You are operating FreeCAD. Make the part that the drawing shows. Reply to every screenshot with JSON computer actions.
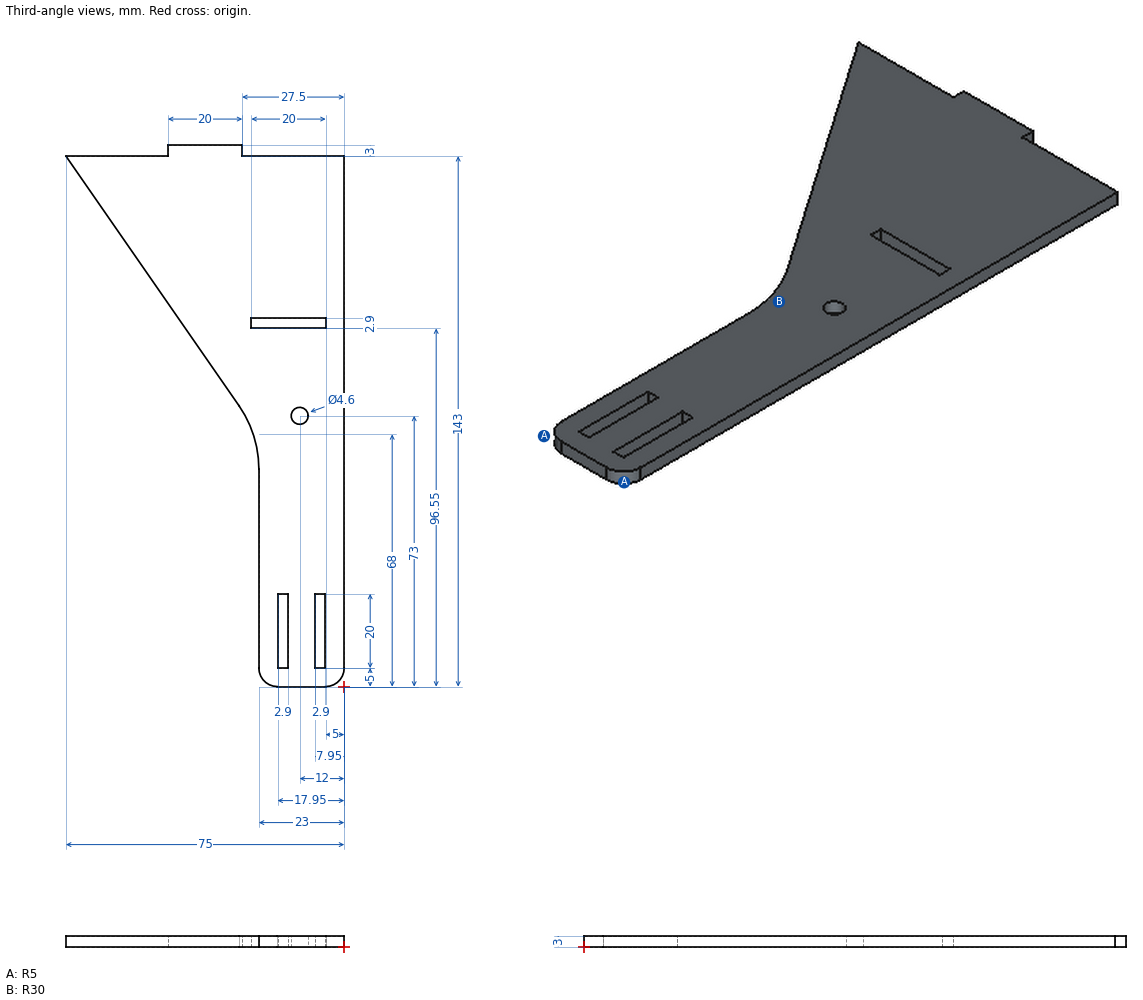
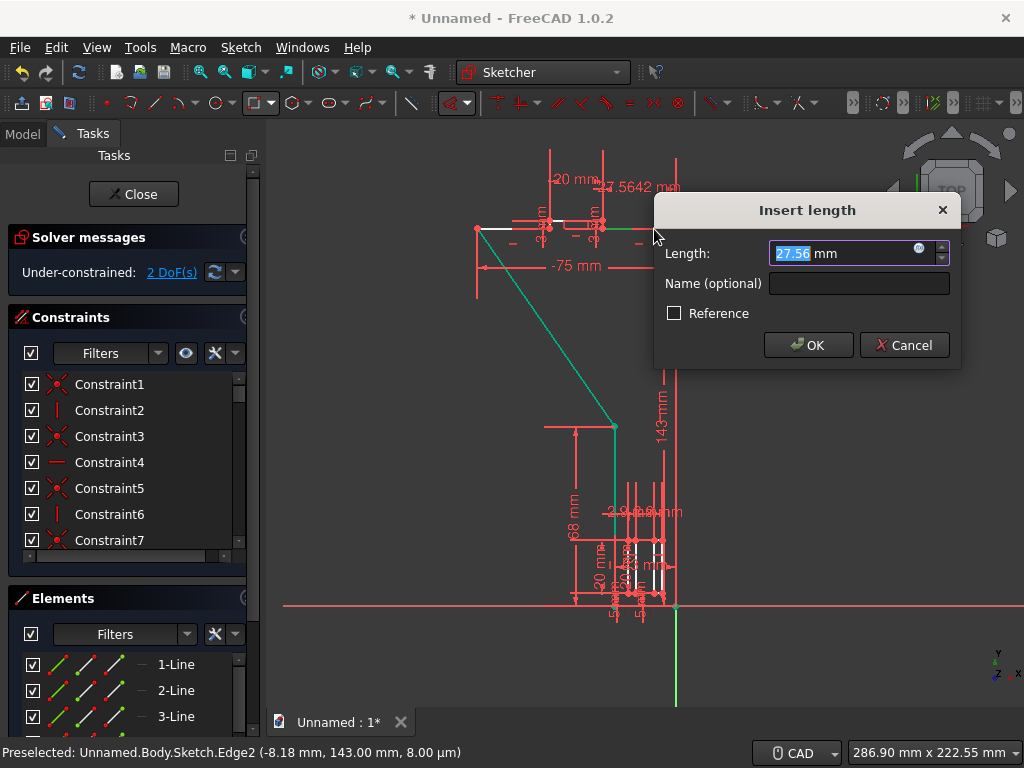
{"action": "type", "text": "27.5"}
{"action": "key", "text": "Return"}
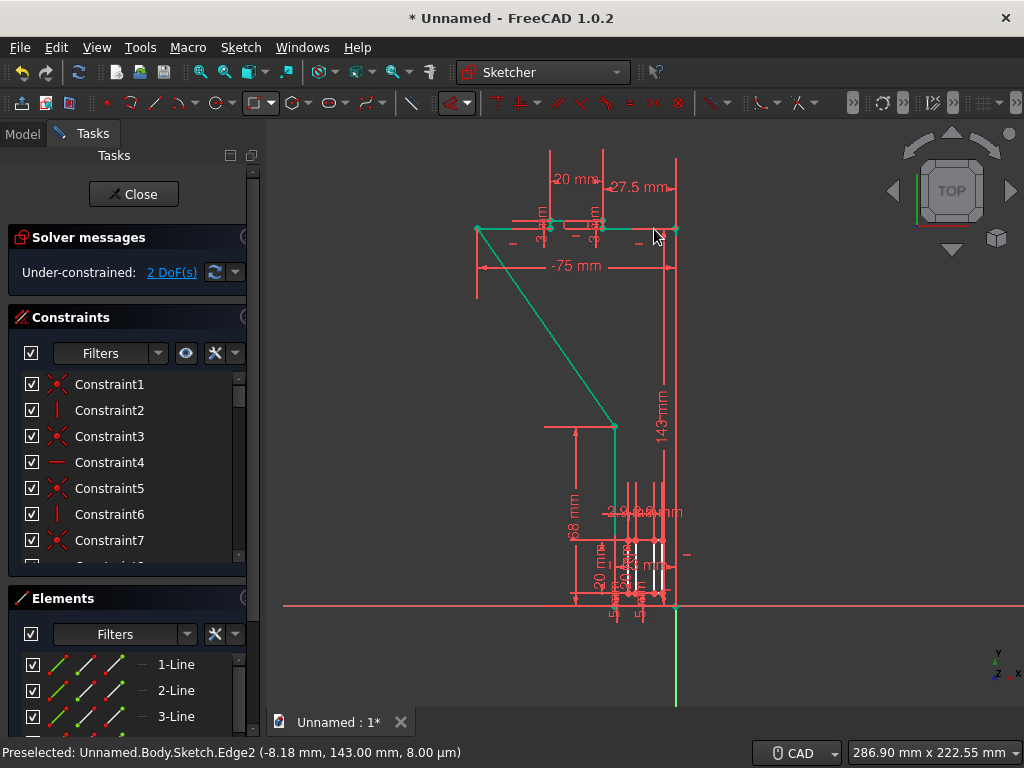
{"action": "scroll", "coordinate": [654, 540], "scroll_direction": "up", "scroll_amount": 4}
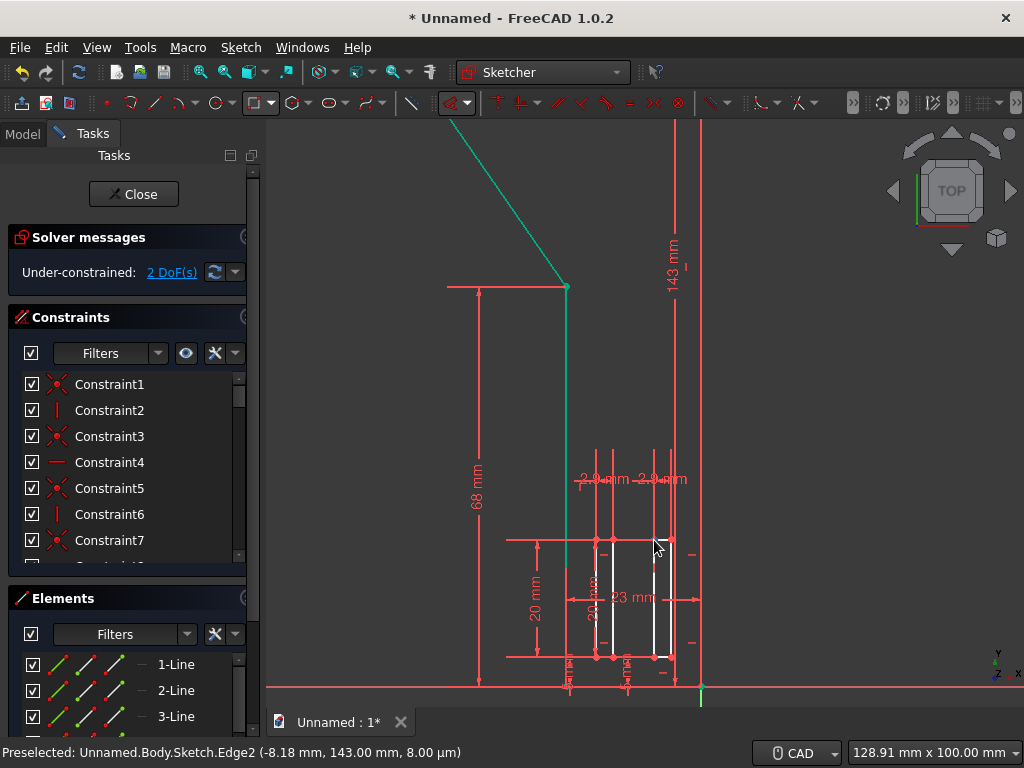
{"action": "left_click", "coordinate": [654, 540]}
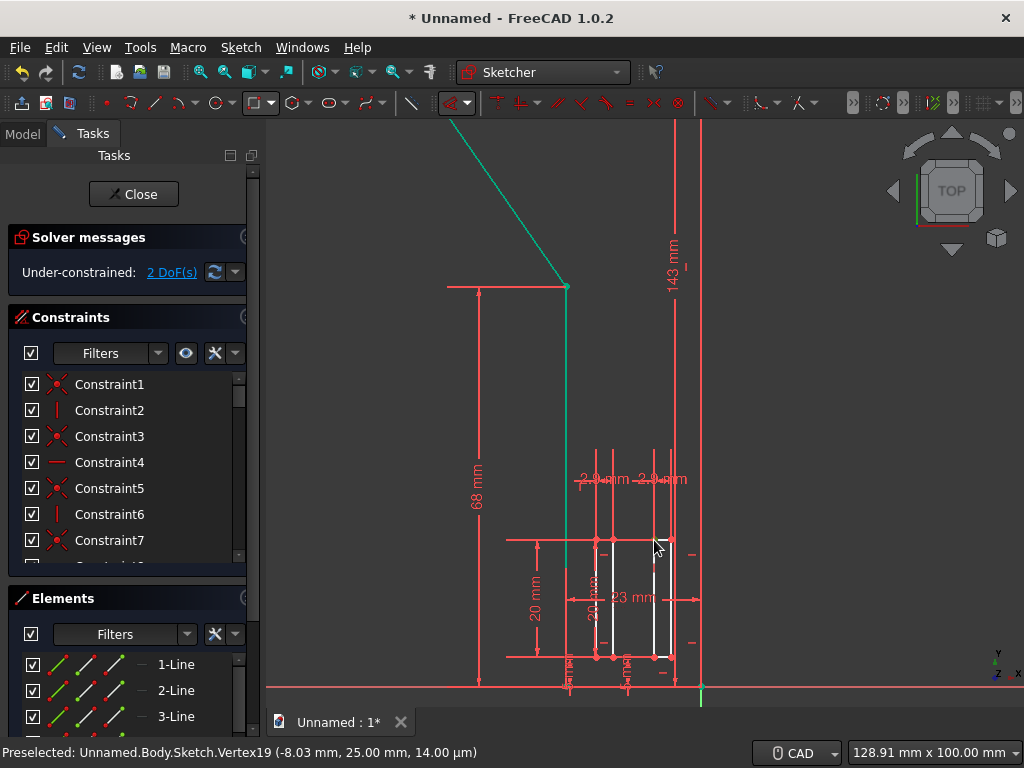
{"action": "key", "text": "l"}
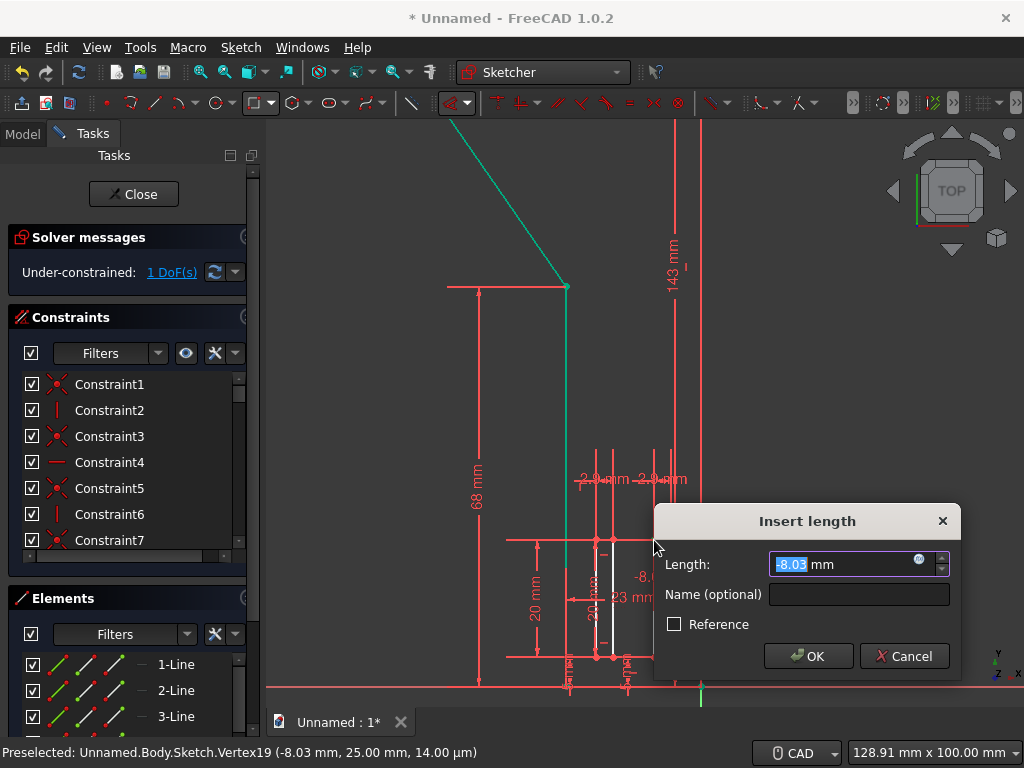
{"action": "type", "text": "-7.95"}
{"action": "key", "text": "Return"}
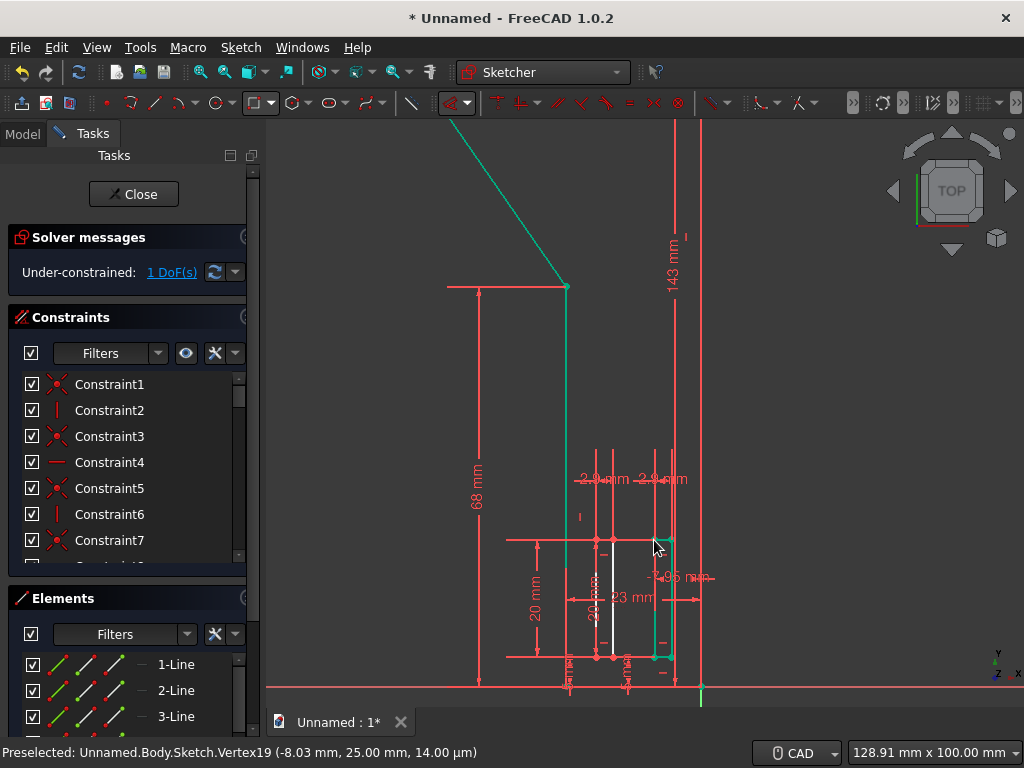
{"action": "left_click", "coordinate": [596, 540]}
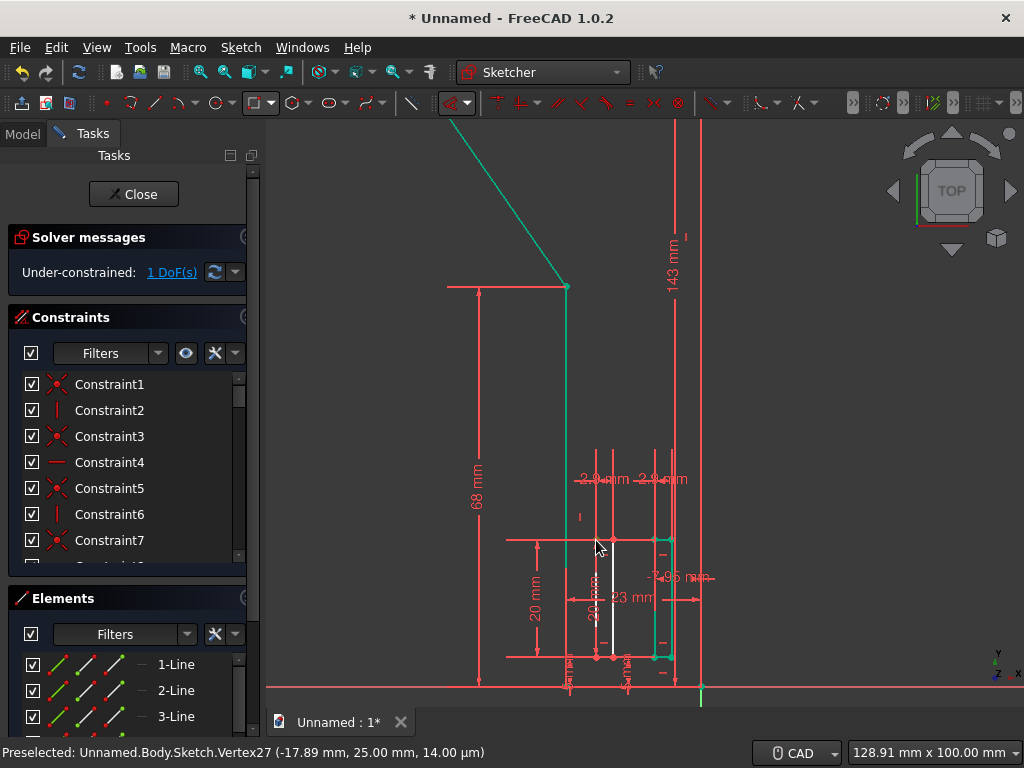
{"action": "left_click", "coordinate": [470, 104]}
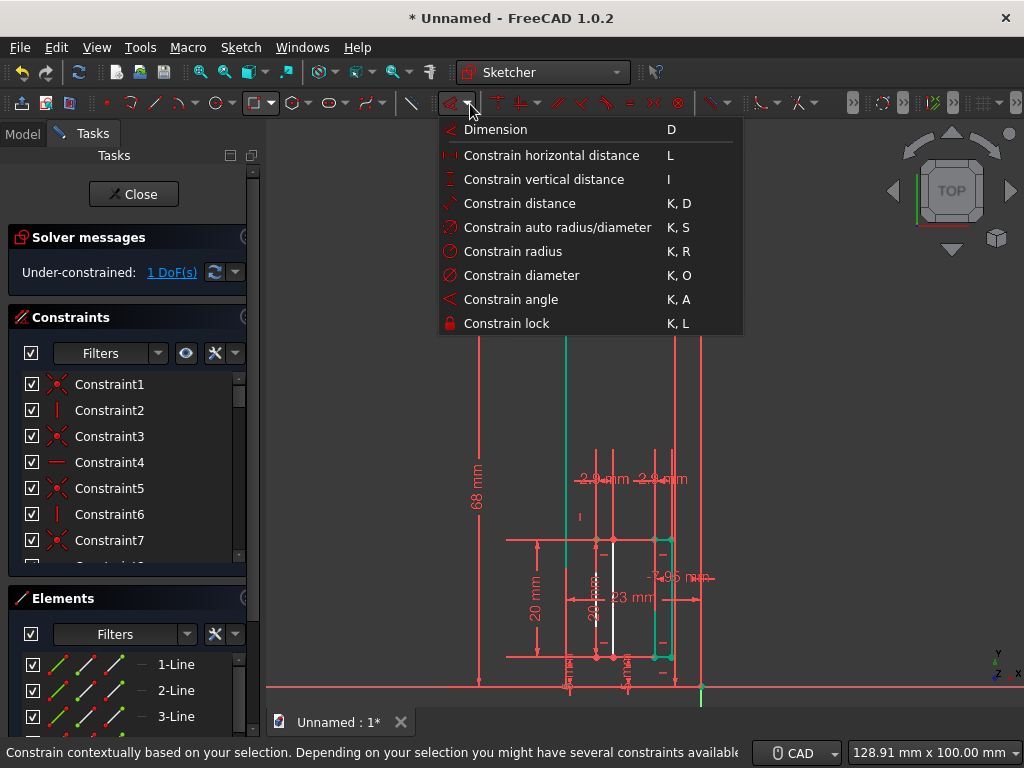
{"action": "left_click", "coordinate": [591, 155]}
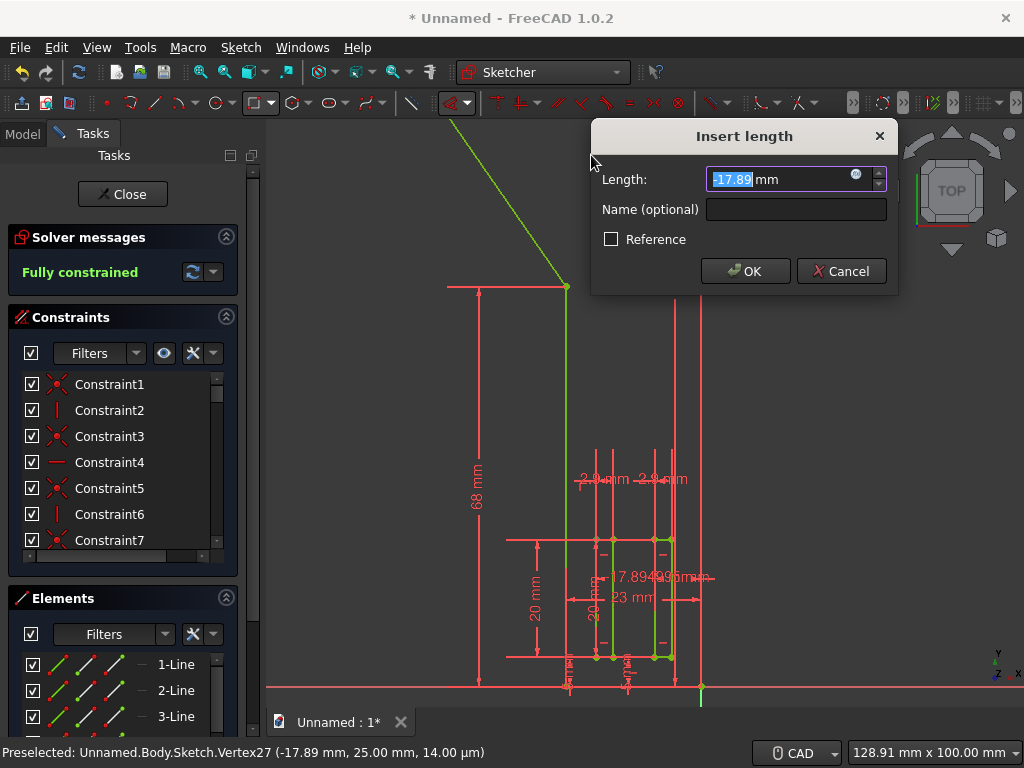
{"action": "type", "text": "-17.95"}
{"action": "key", "text": "Return"}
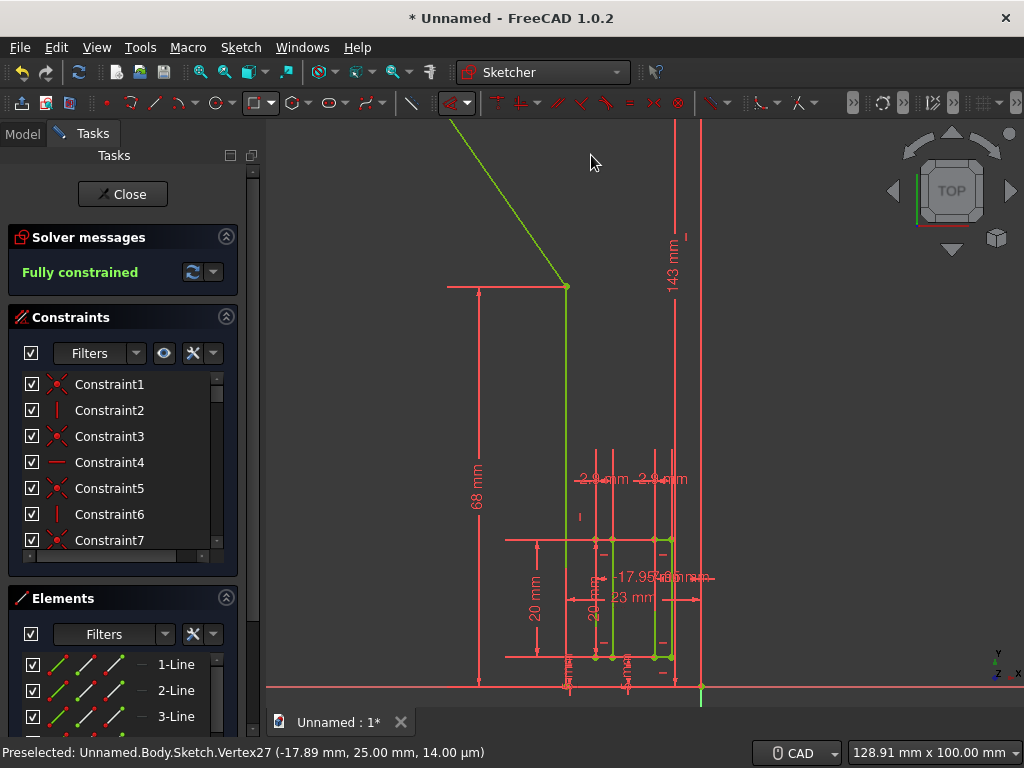
{"action": "left_click", "coordinate": [123, 194]}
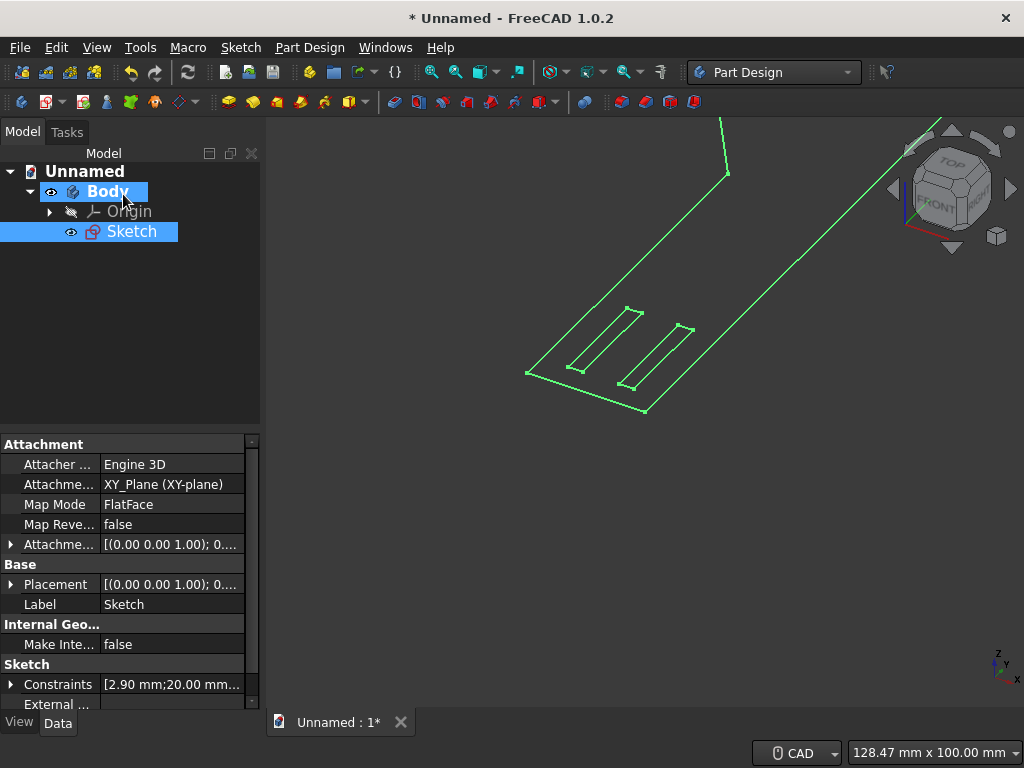
{"action": "left_click", "coordinate": [230, 102]}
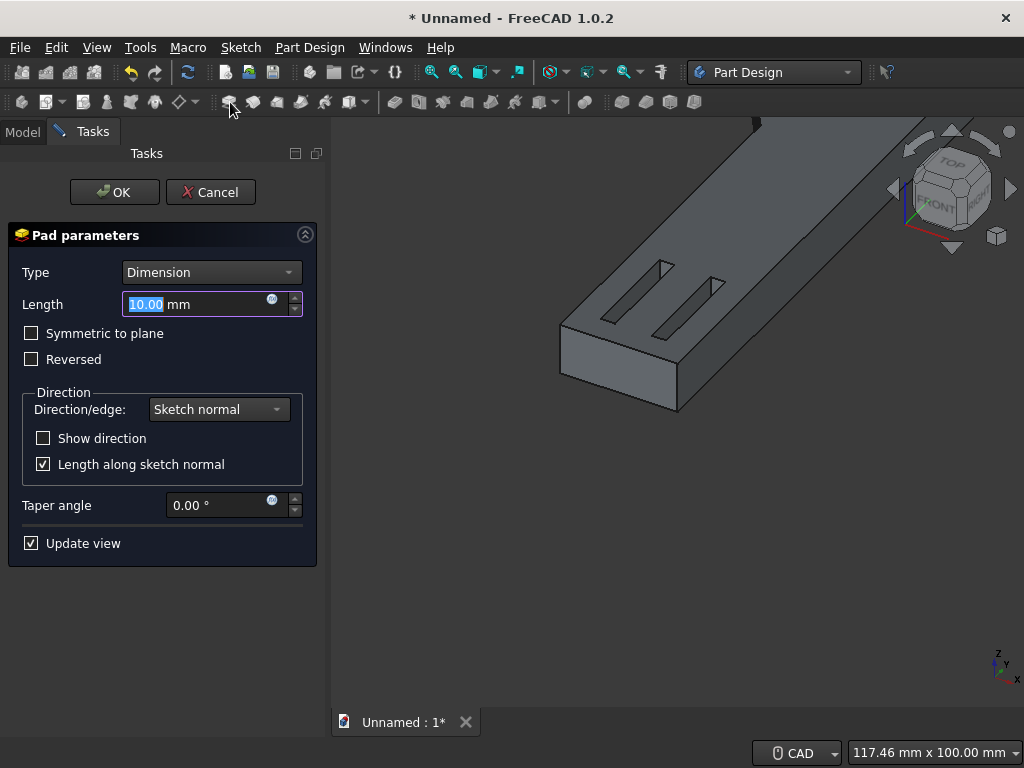
{"action": "type", "text": "3"}
{"action": "key", "text": "Tab"}